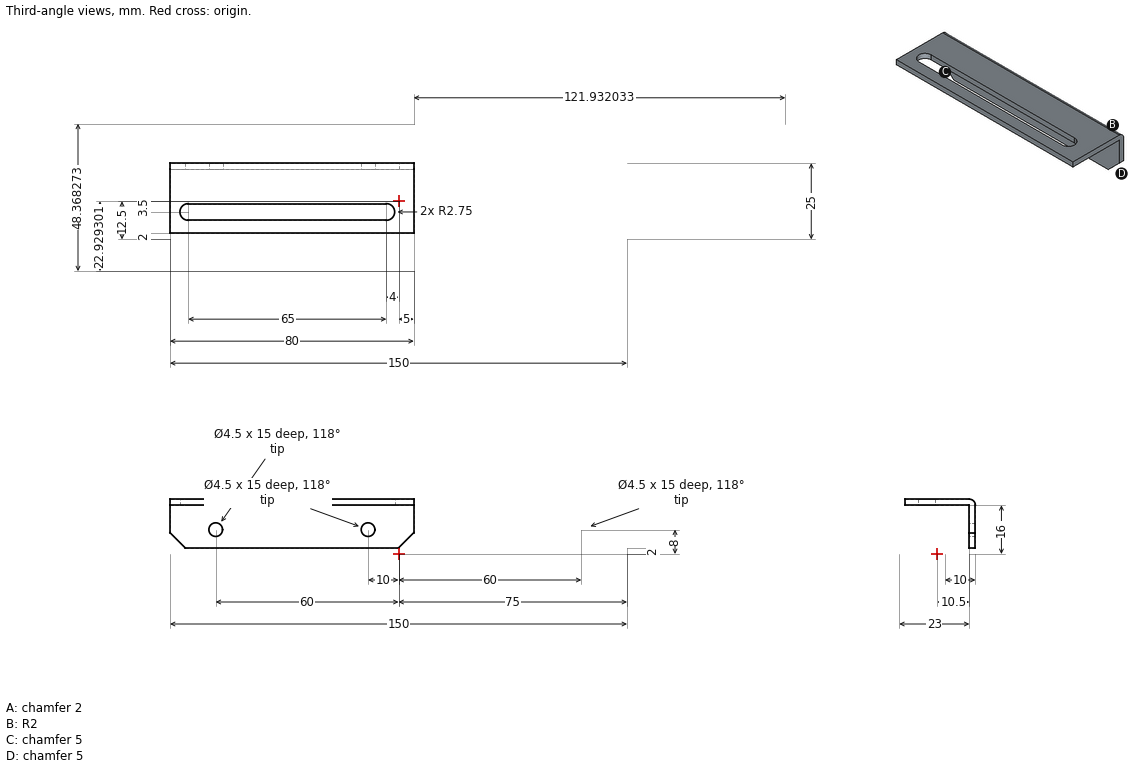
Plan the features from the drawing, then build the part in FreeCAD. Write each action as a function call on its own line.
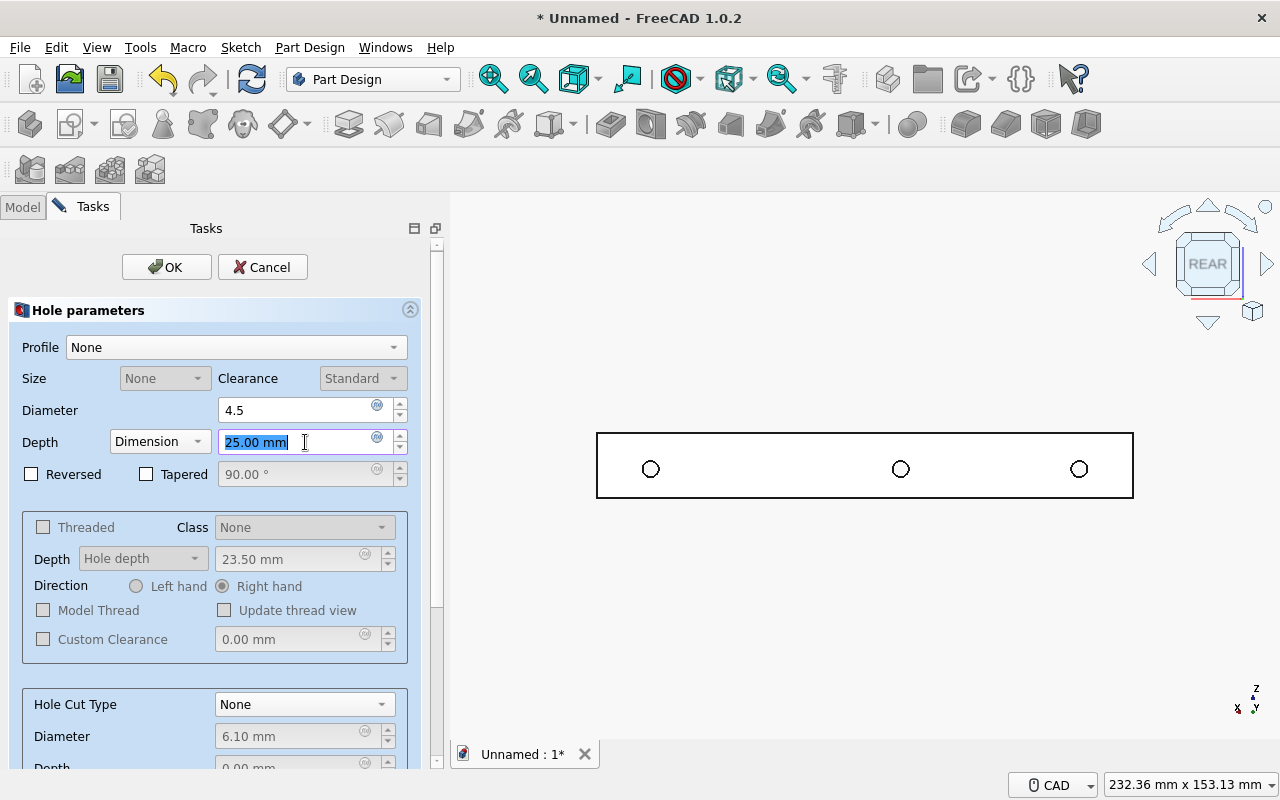
text(15)
key(Tab)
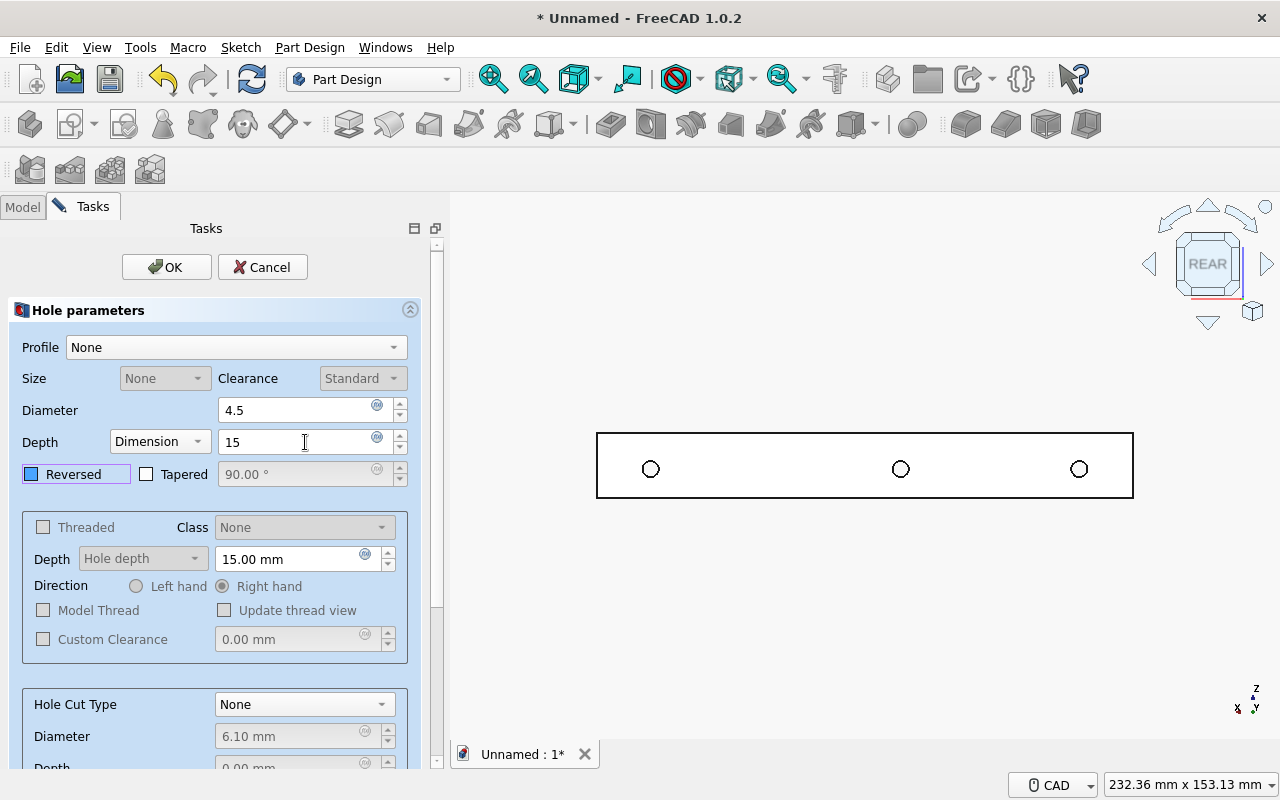
click(167, 267)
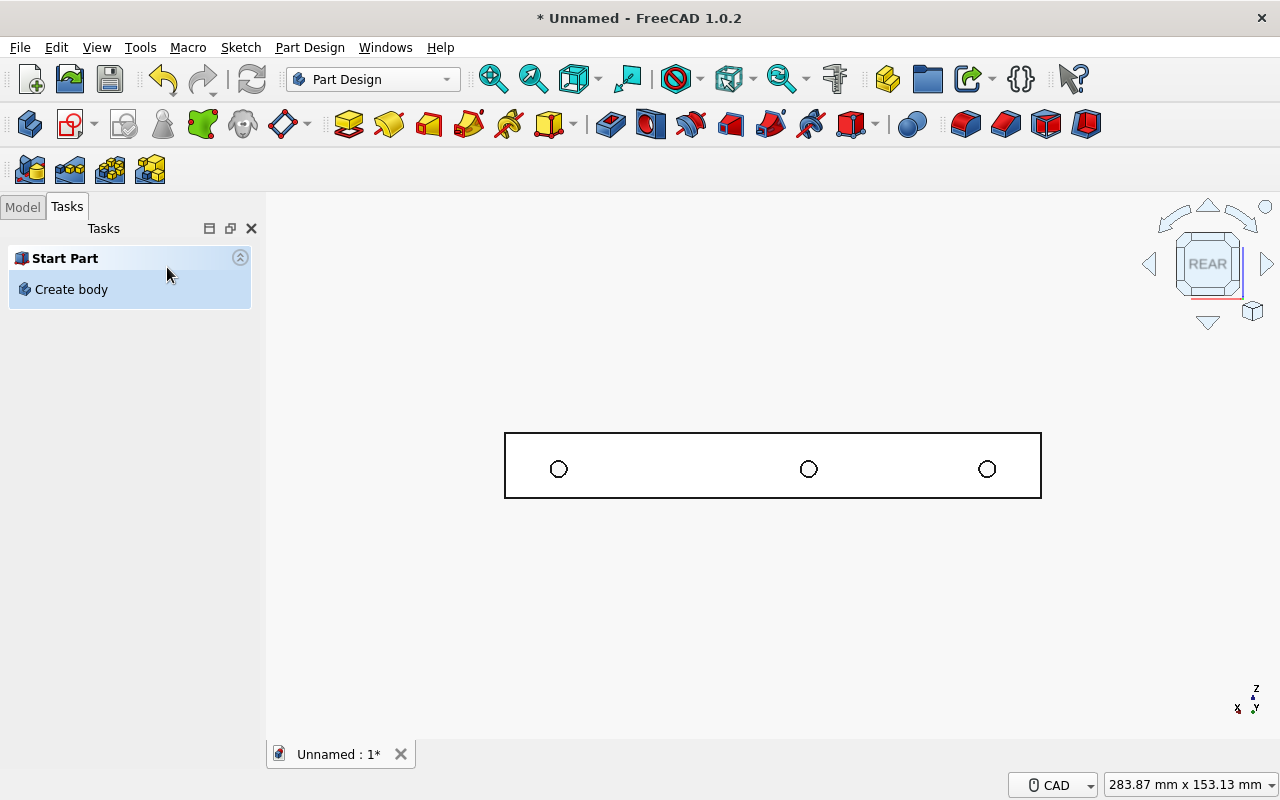
scroll(505, 436, up, 9)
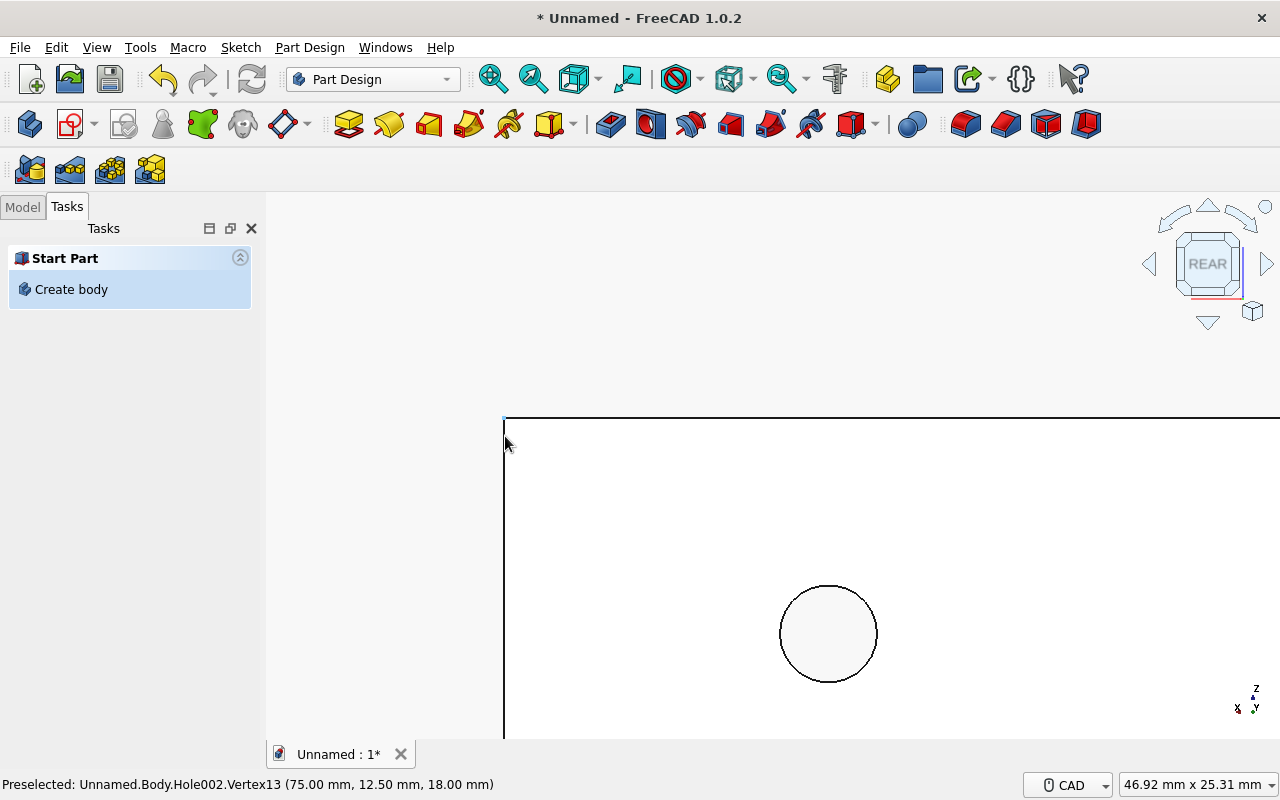
click(494, 80)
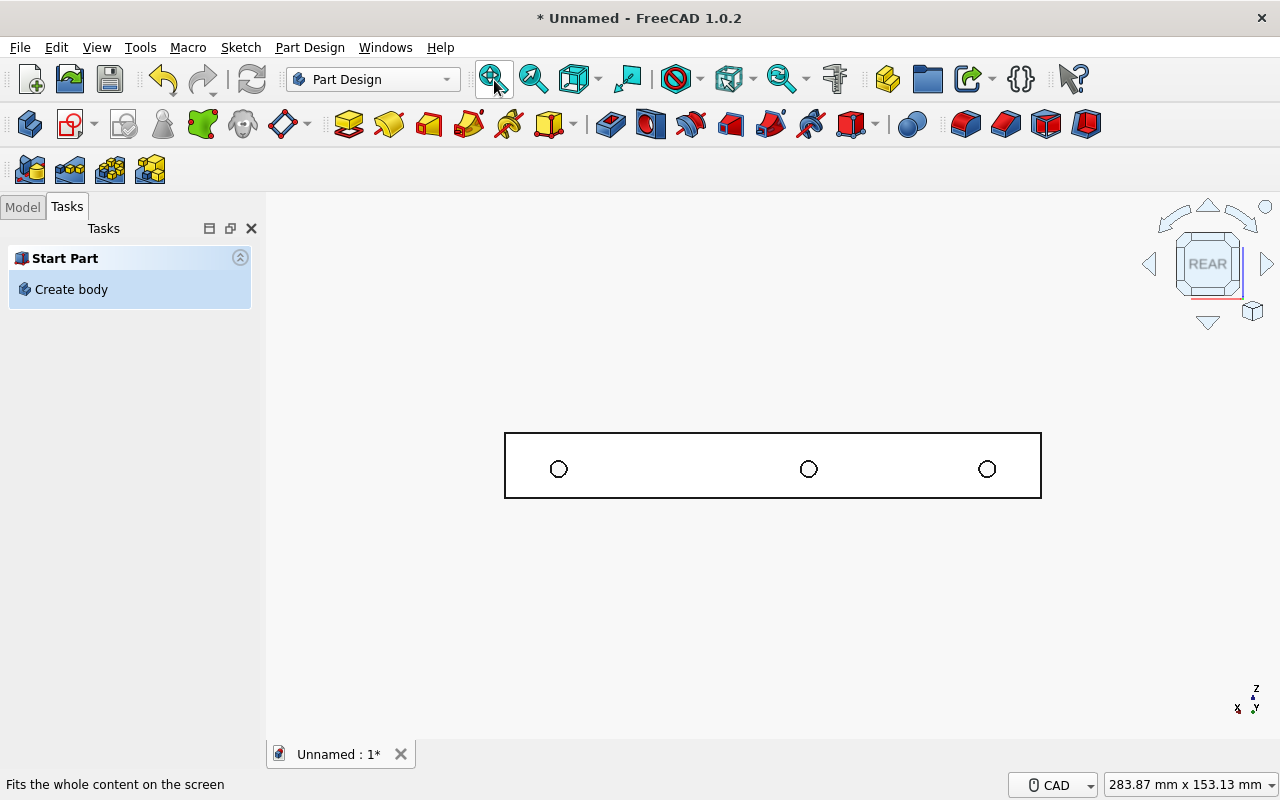
key(0)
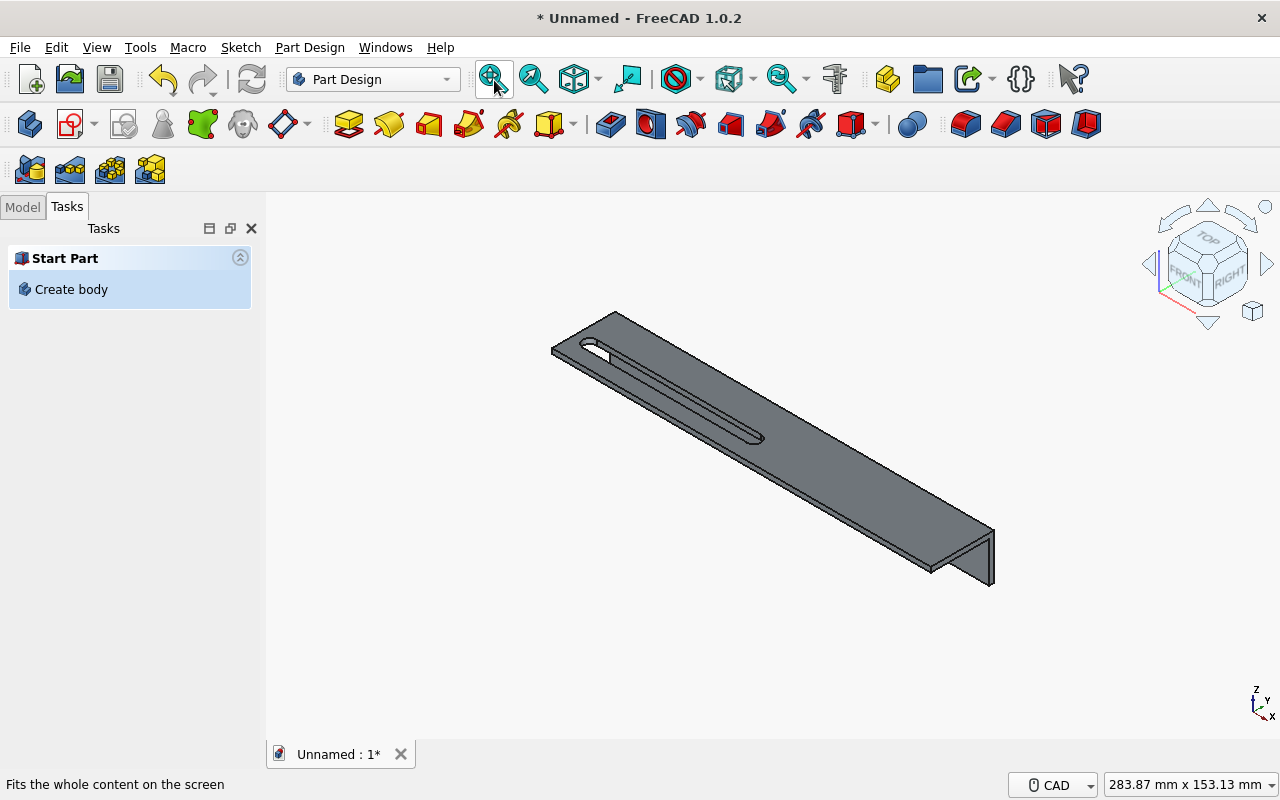
scroll(931, 569, up, 9)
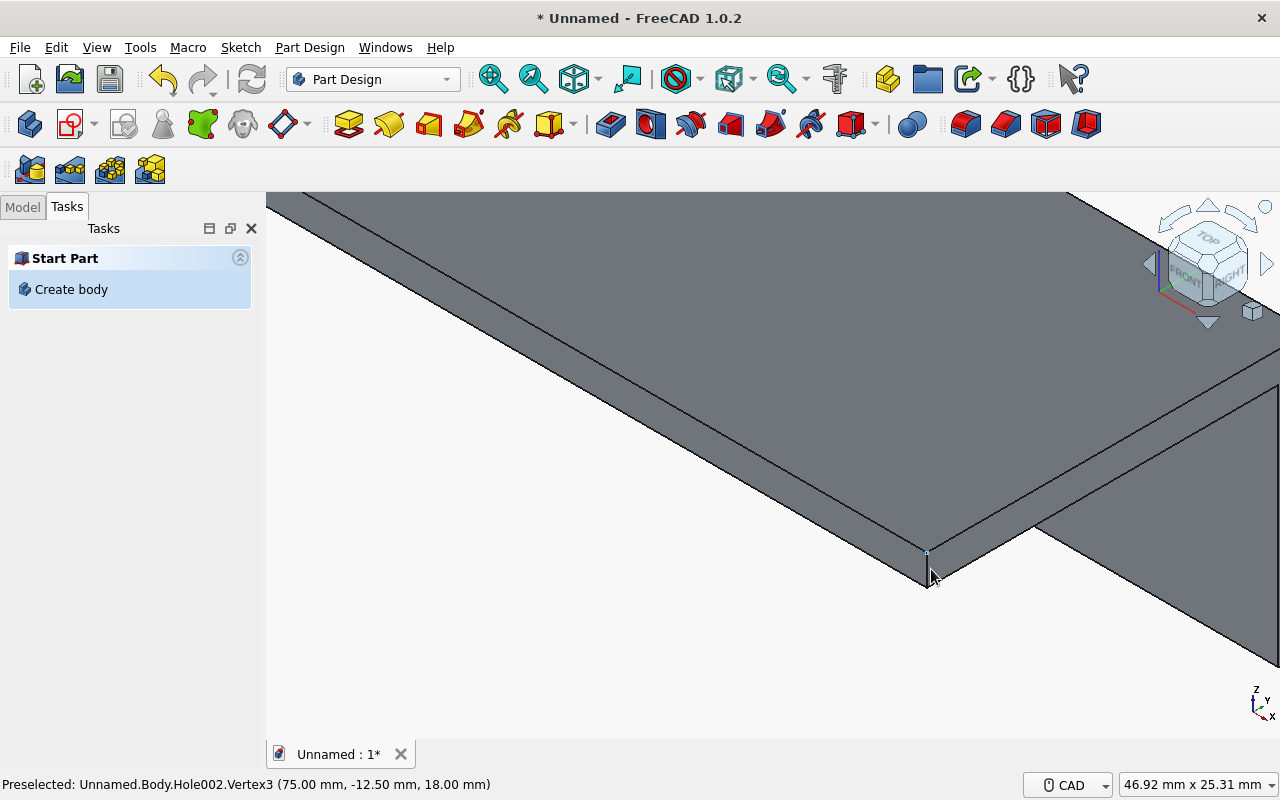
click(927, 569)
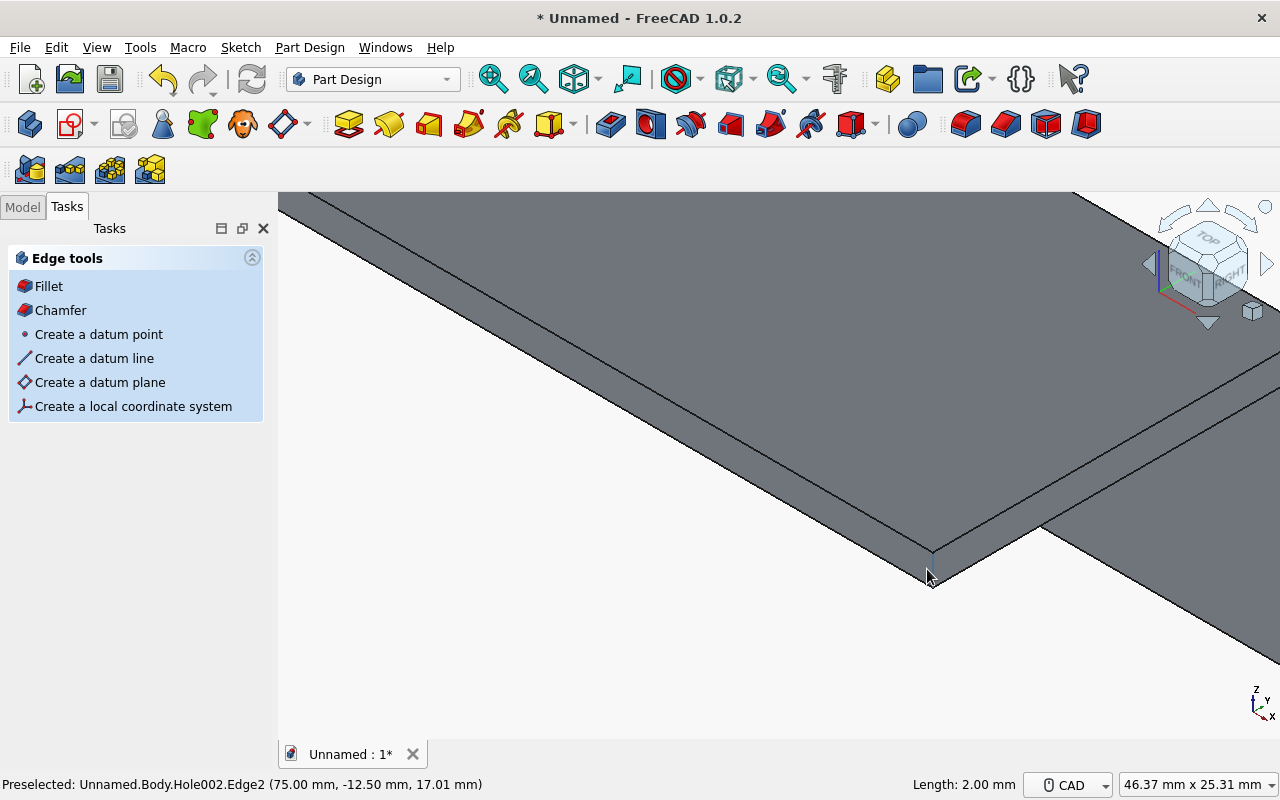
click(1006, 124)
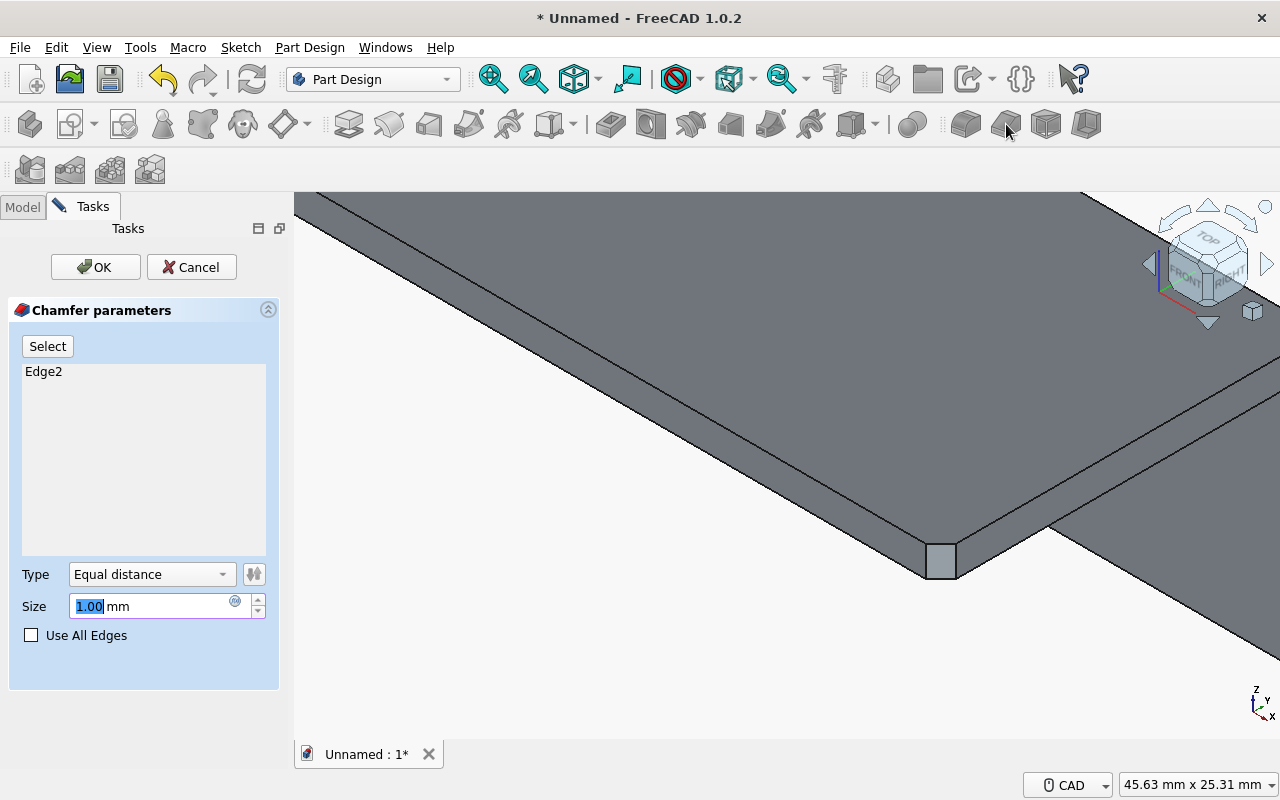
text(2)
key(Tab)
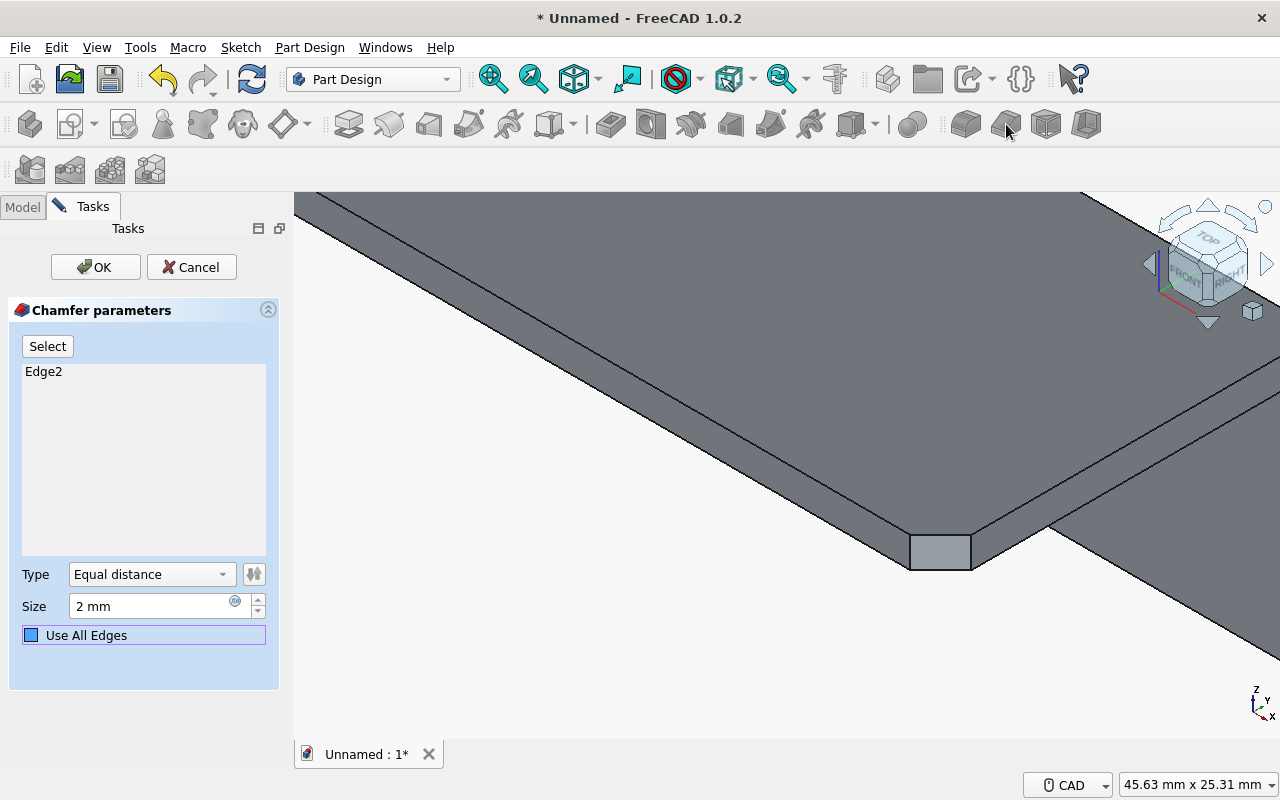
click(96, 267)